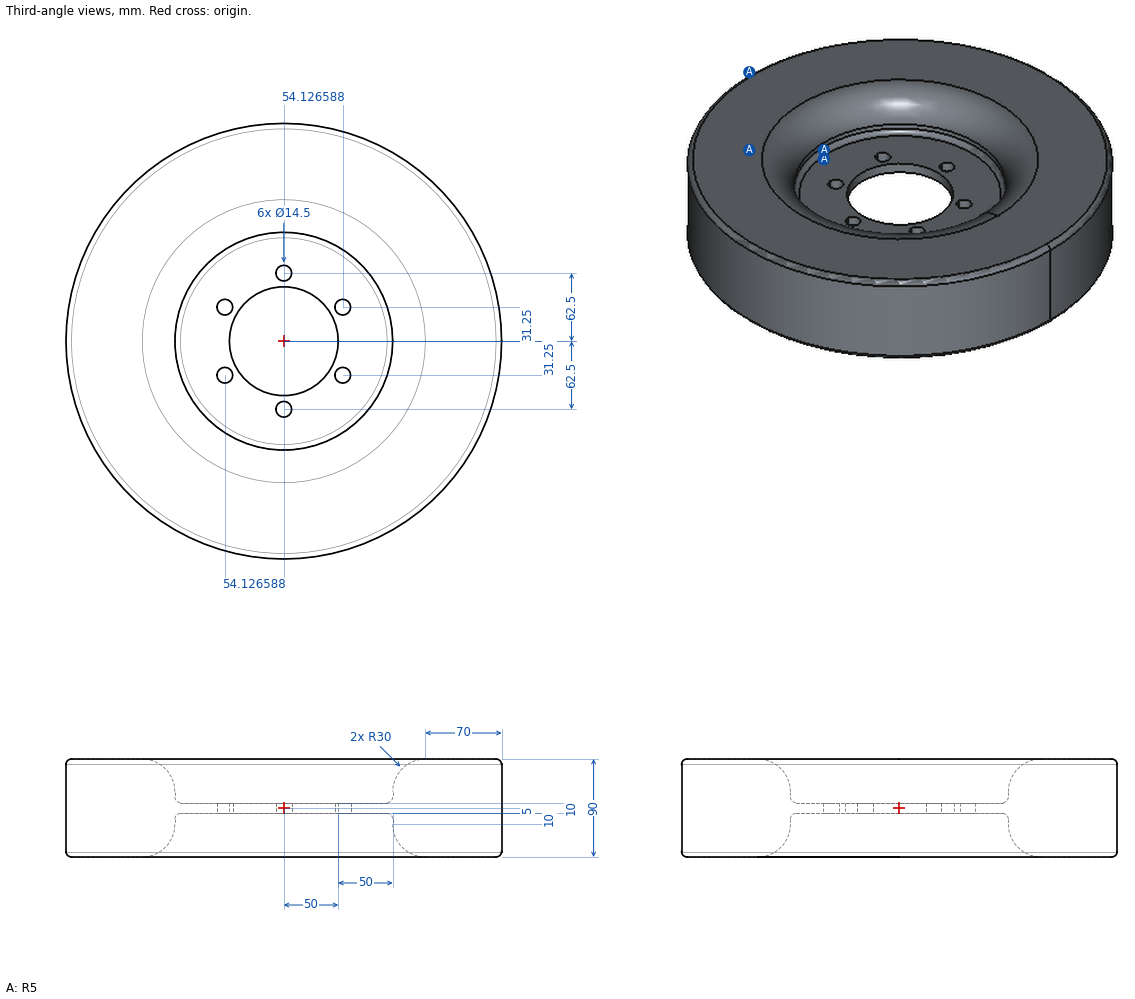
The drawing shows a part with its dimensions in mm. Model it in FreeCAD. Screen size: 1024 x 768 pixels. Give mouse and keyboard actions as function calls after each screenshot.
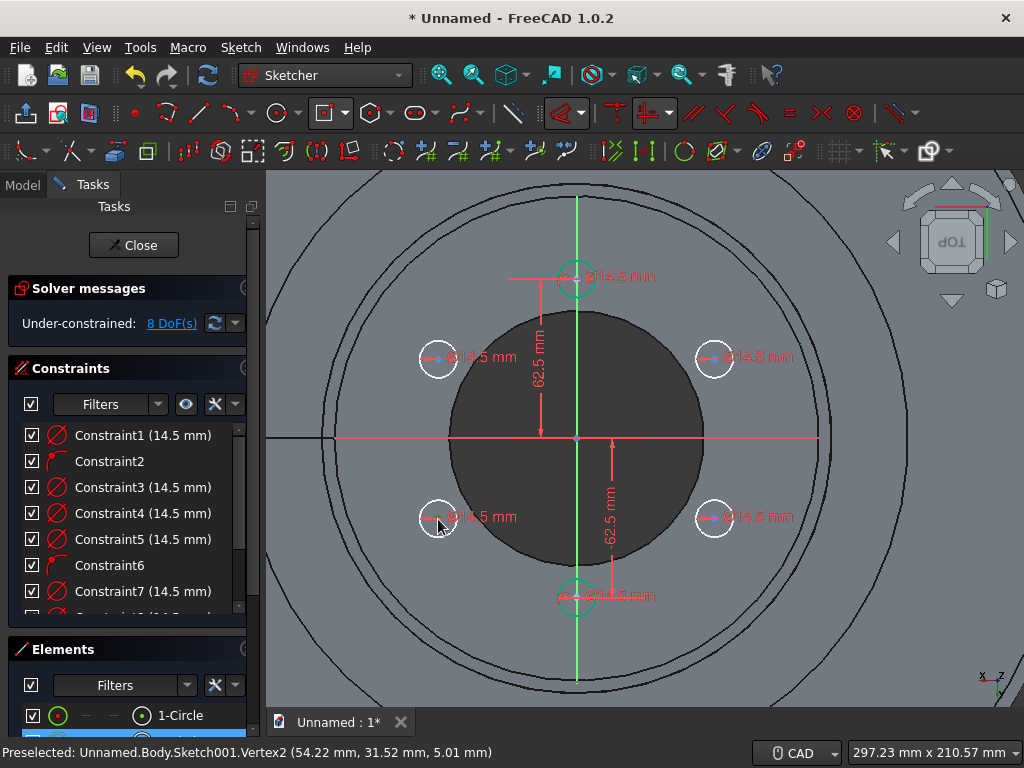
key(i)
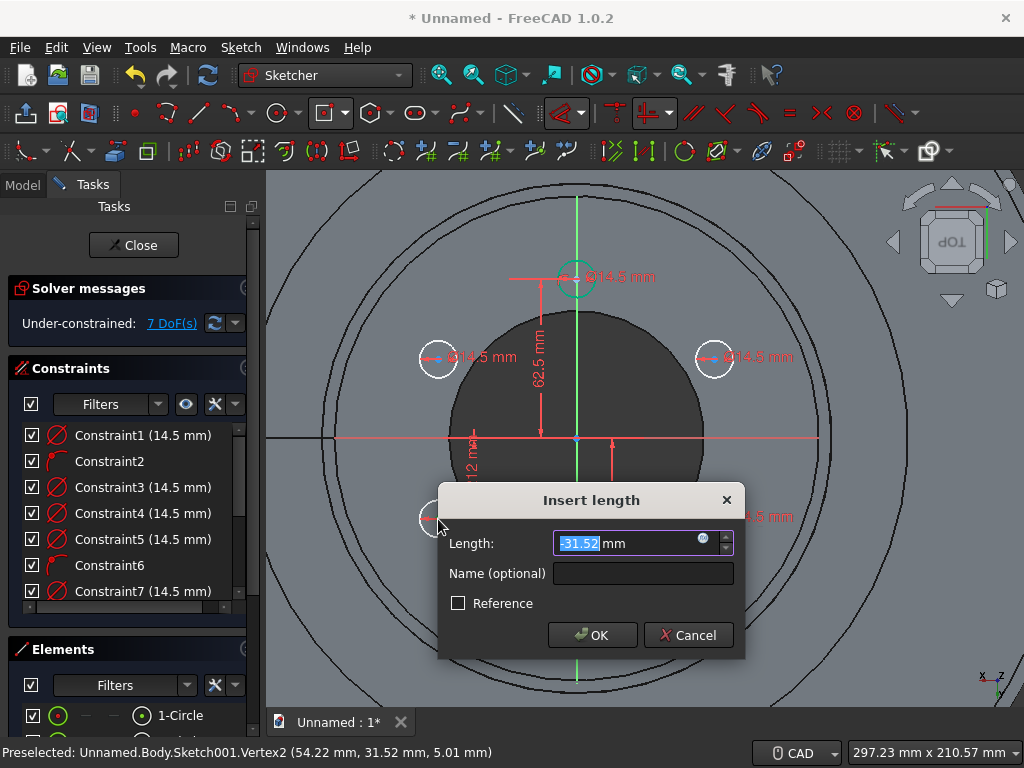
text(-31.25)
key(Return)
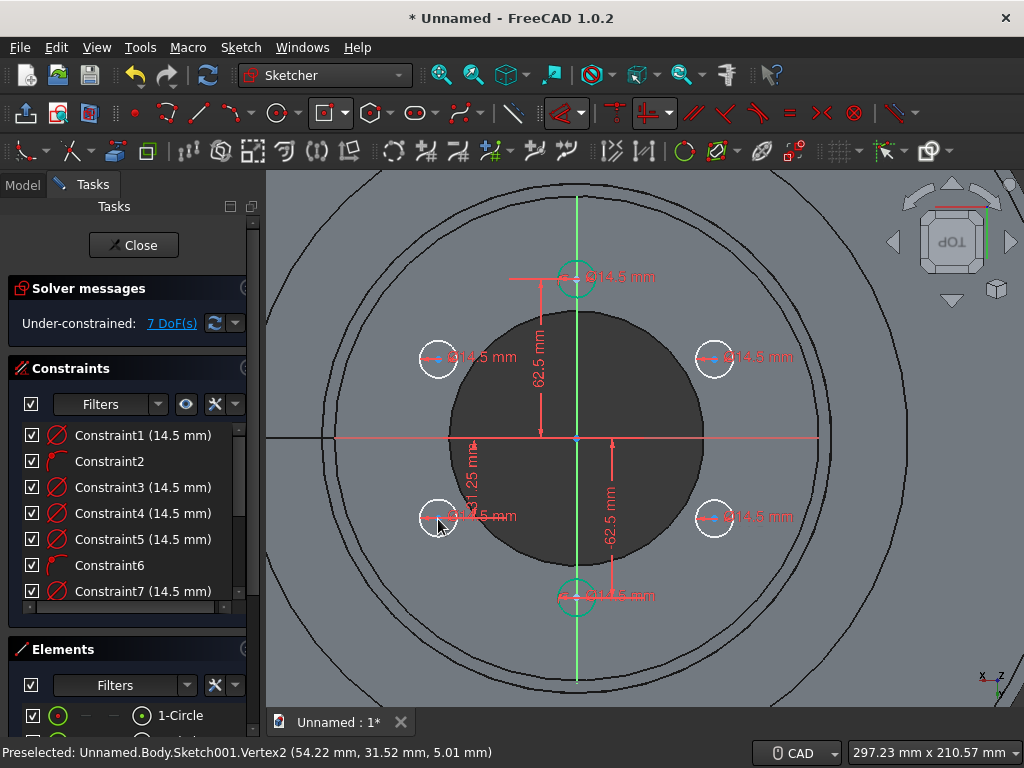
click(438, 359)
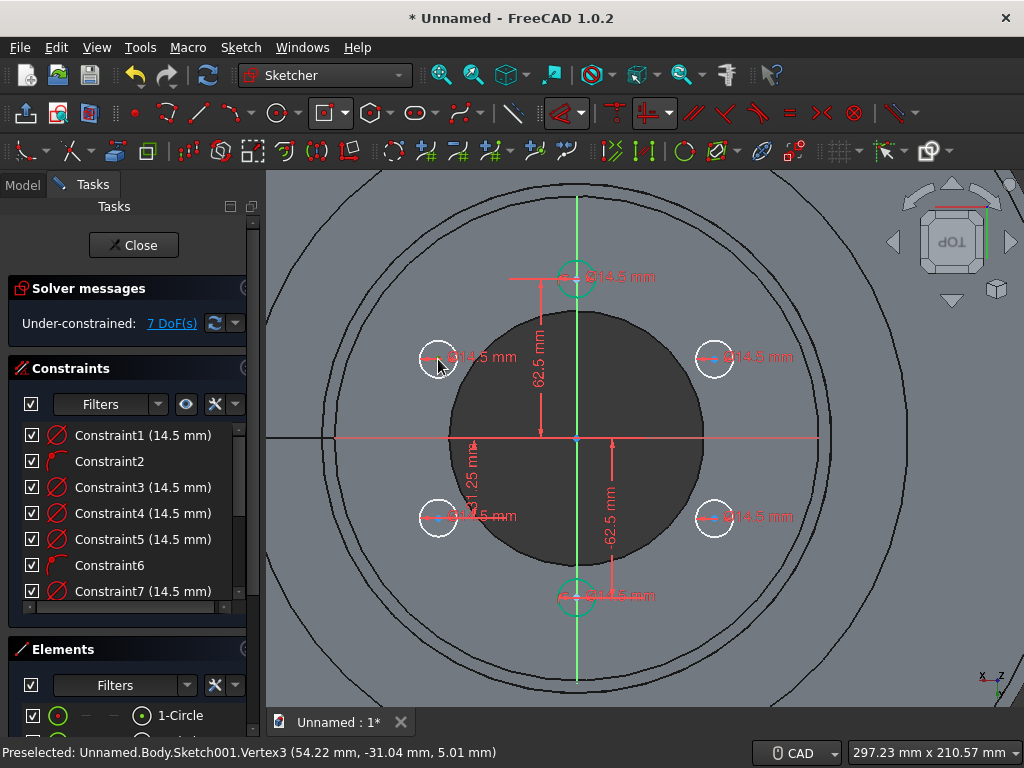
key(i)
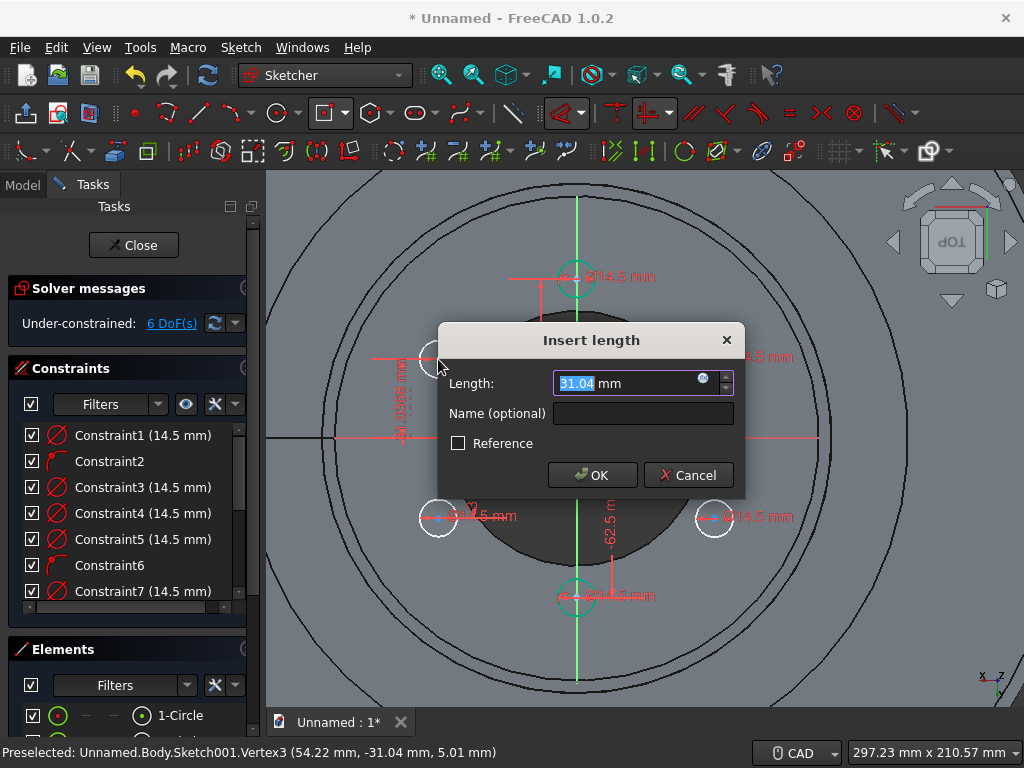
text(31.25)
key(Return)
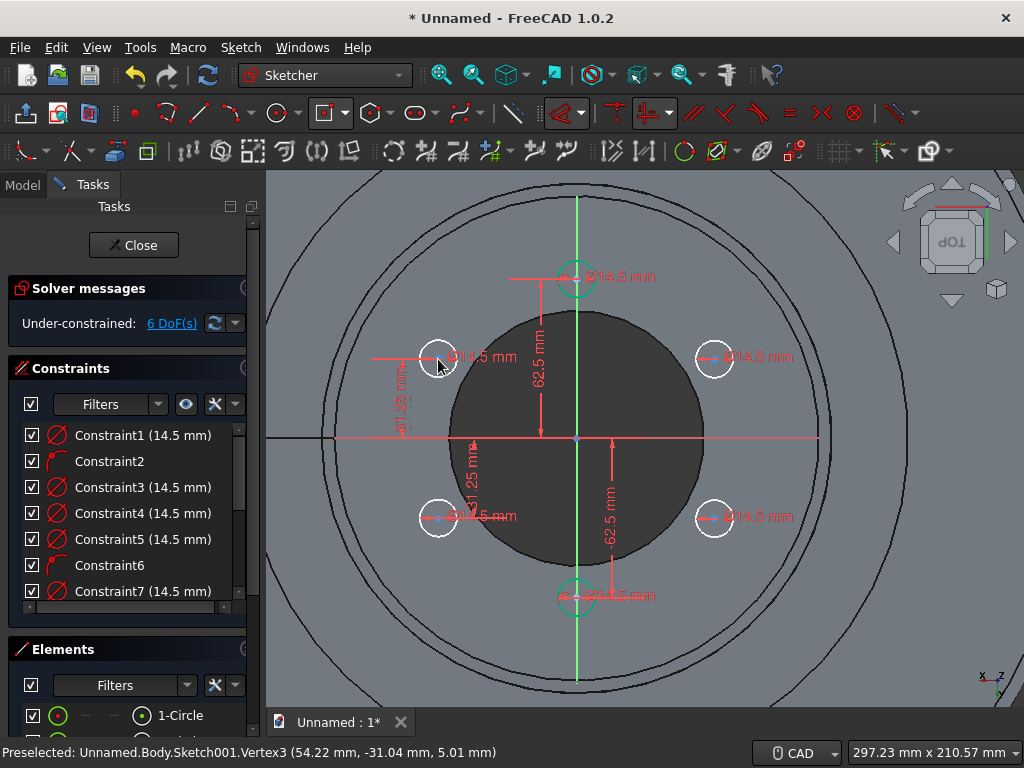
click(715, 359)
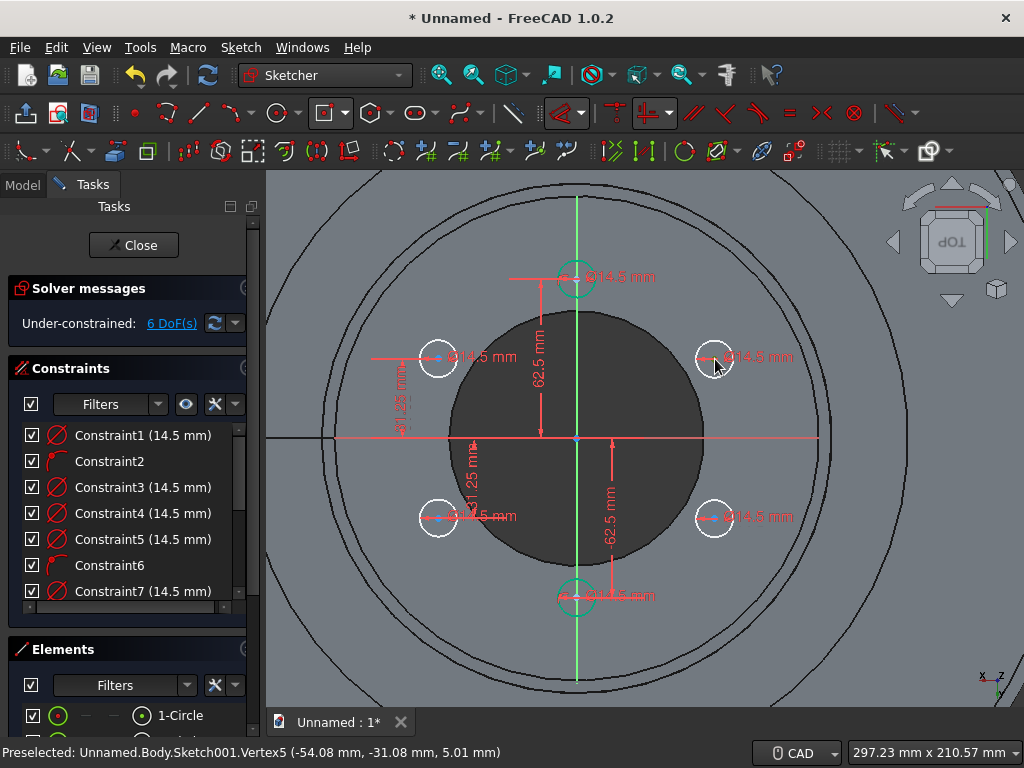
click(584, 114)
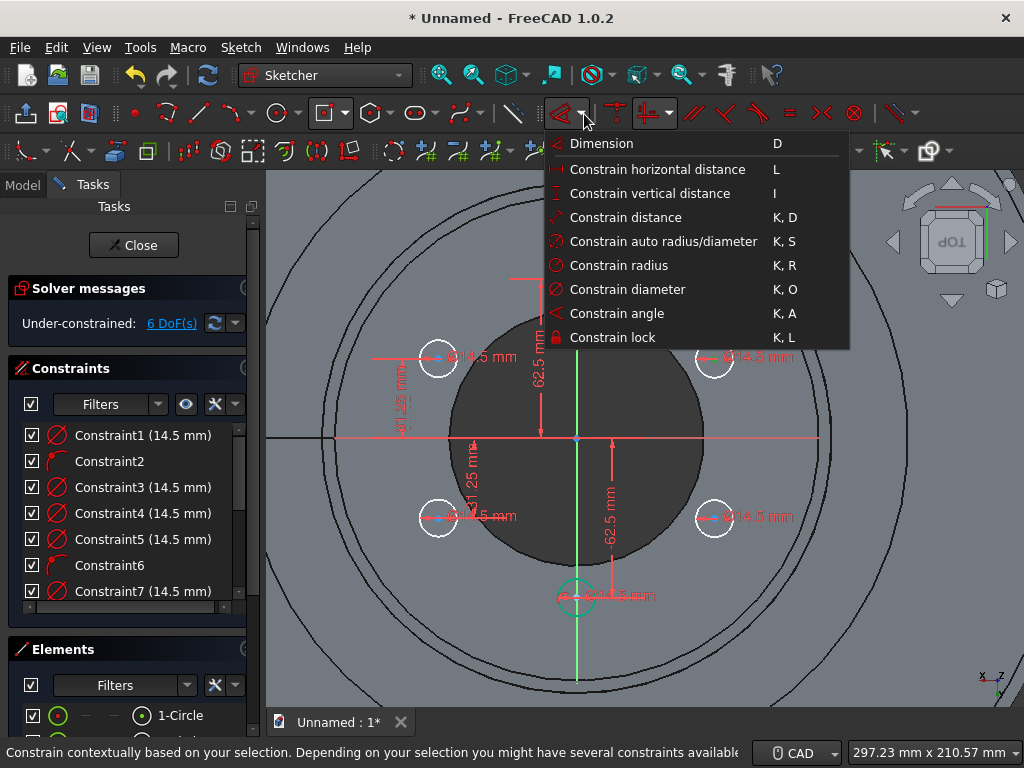
click(697, 193)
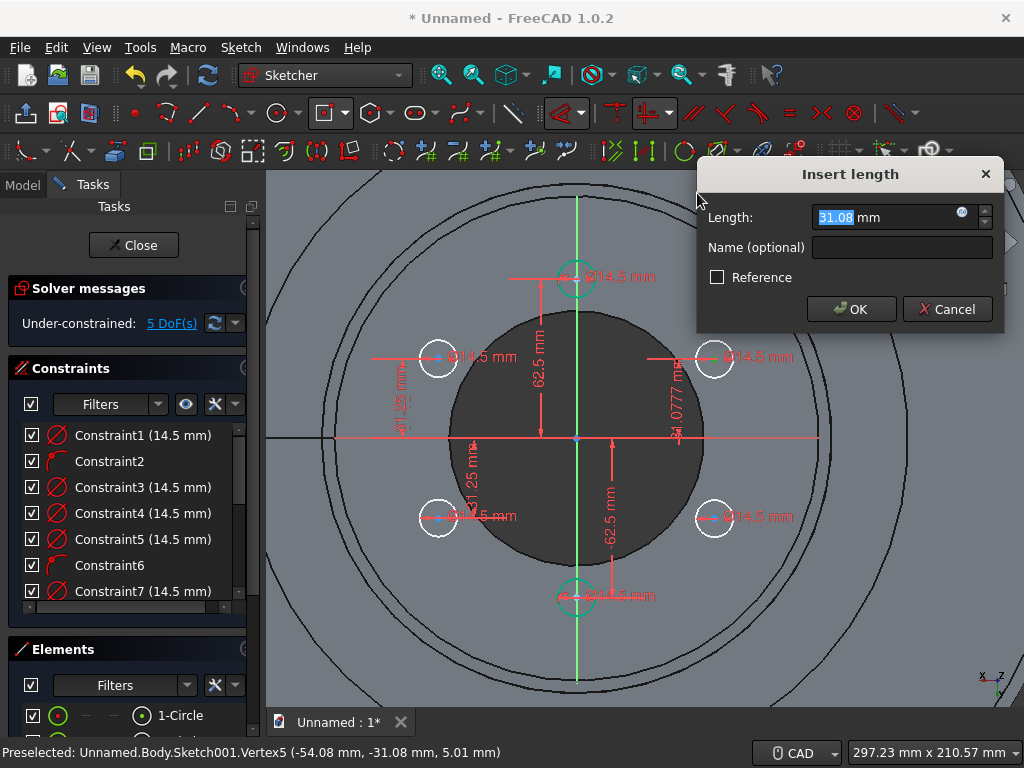
text(31.25)
key(Return)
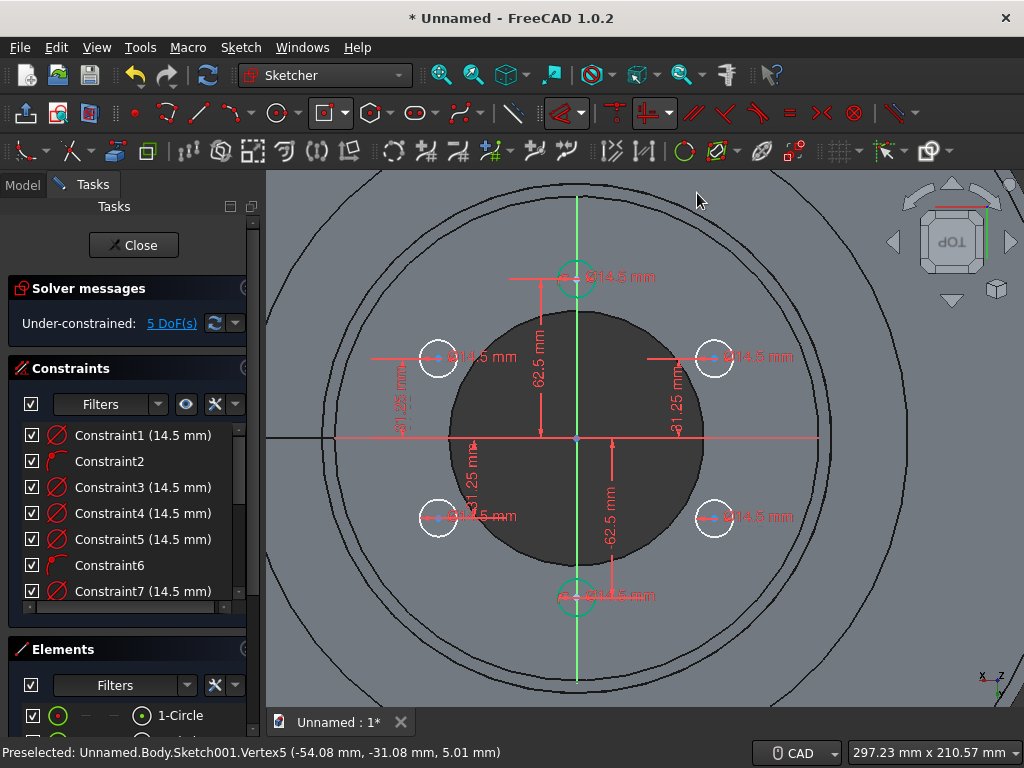
click(715, 519)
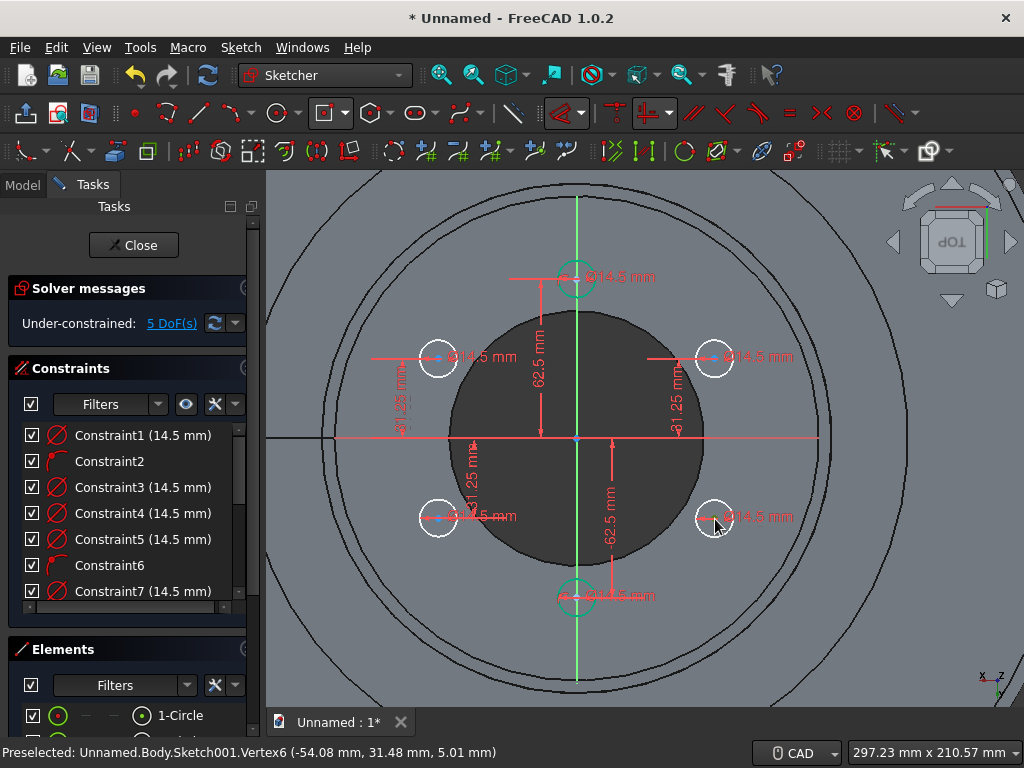
click(584, 114)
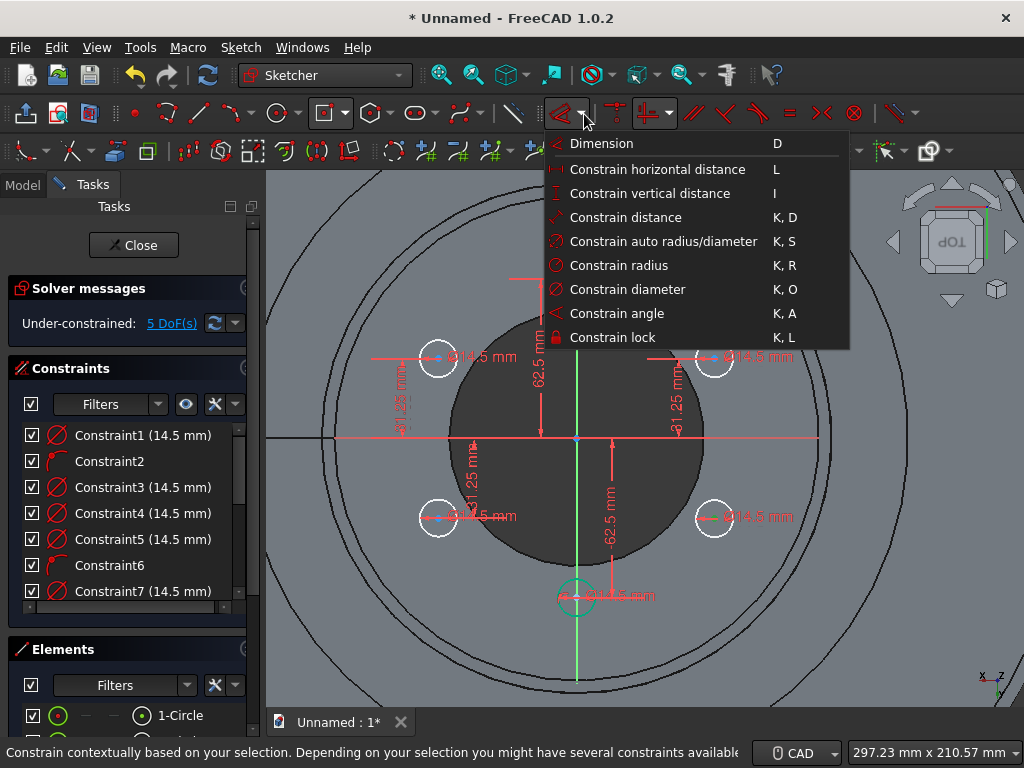
click(697, 193)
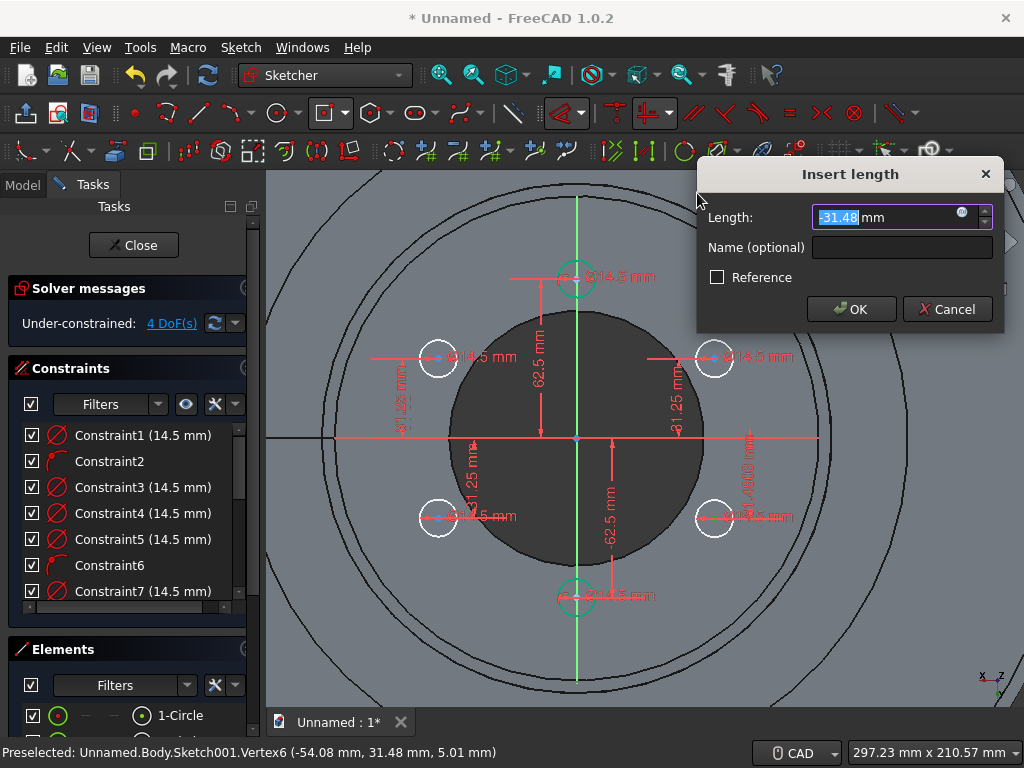
text(-31.25)
key(Return)